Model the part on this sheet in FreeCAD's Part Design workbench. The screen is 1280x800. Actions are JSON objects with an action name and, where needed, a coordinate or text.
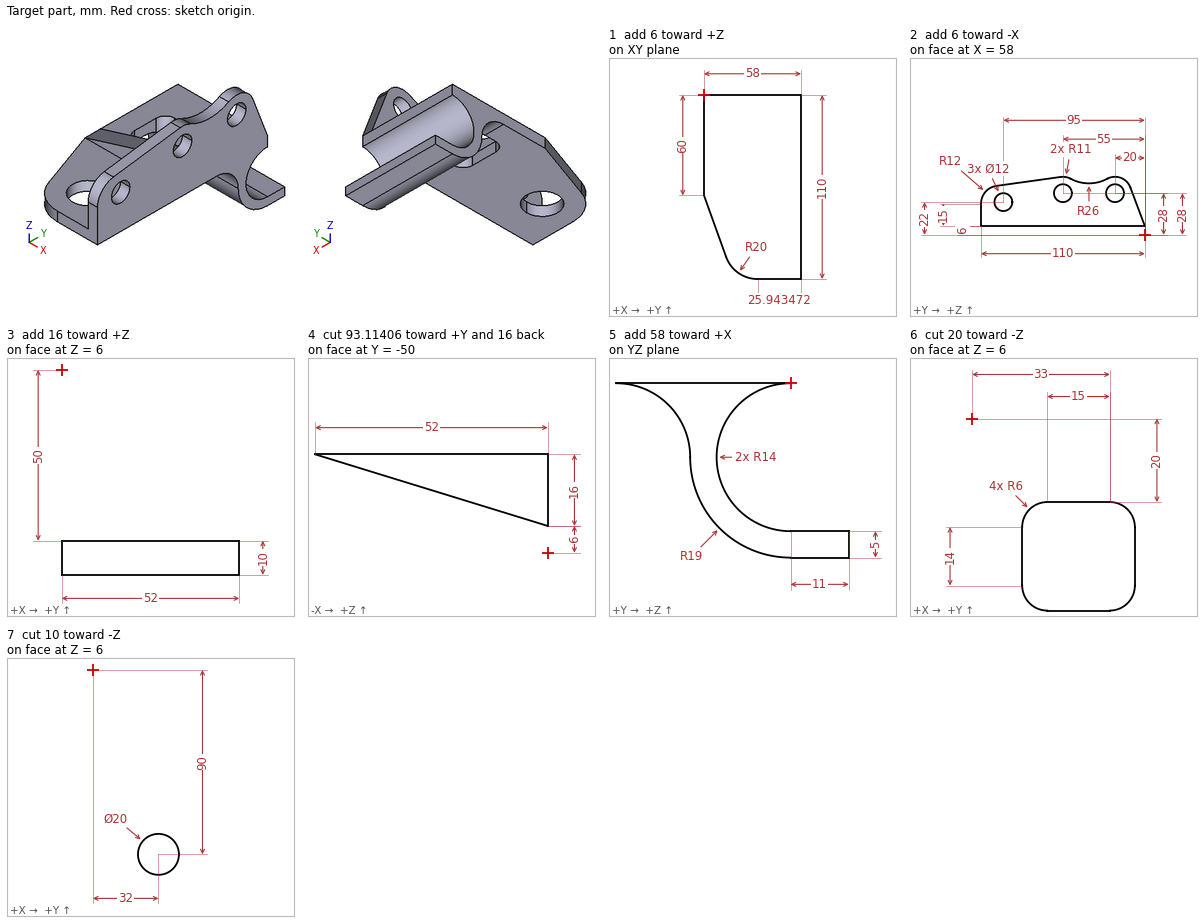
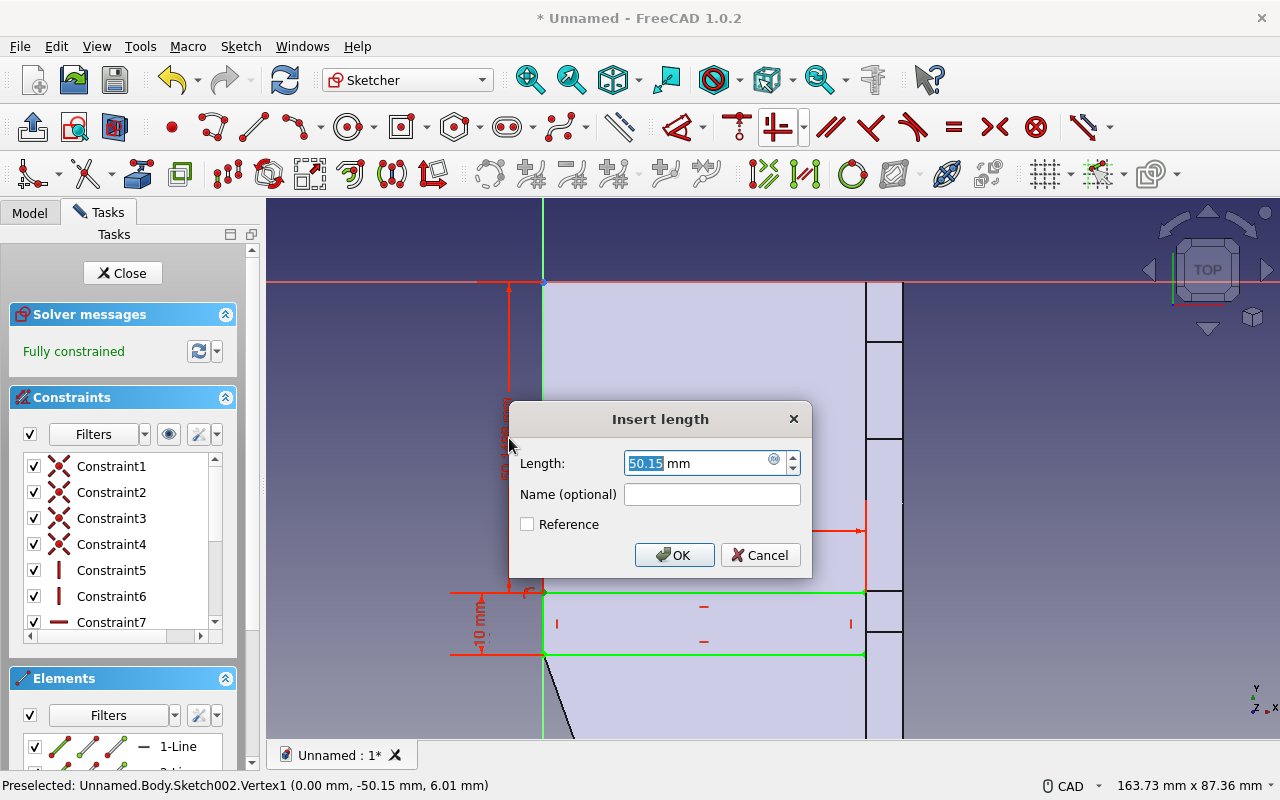
{"action": "type", "text": "50"}
{"action": "key", "text": "Return"}
{"action": "key", "text": "Escape"}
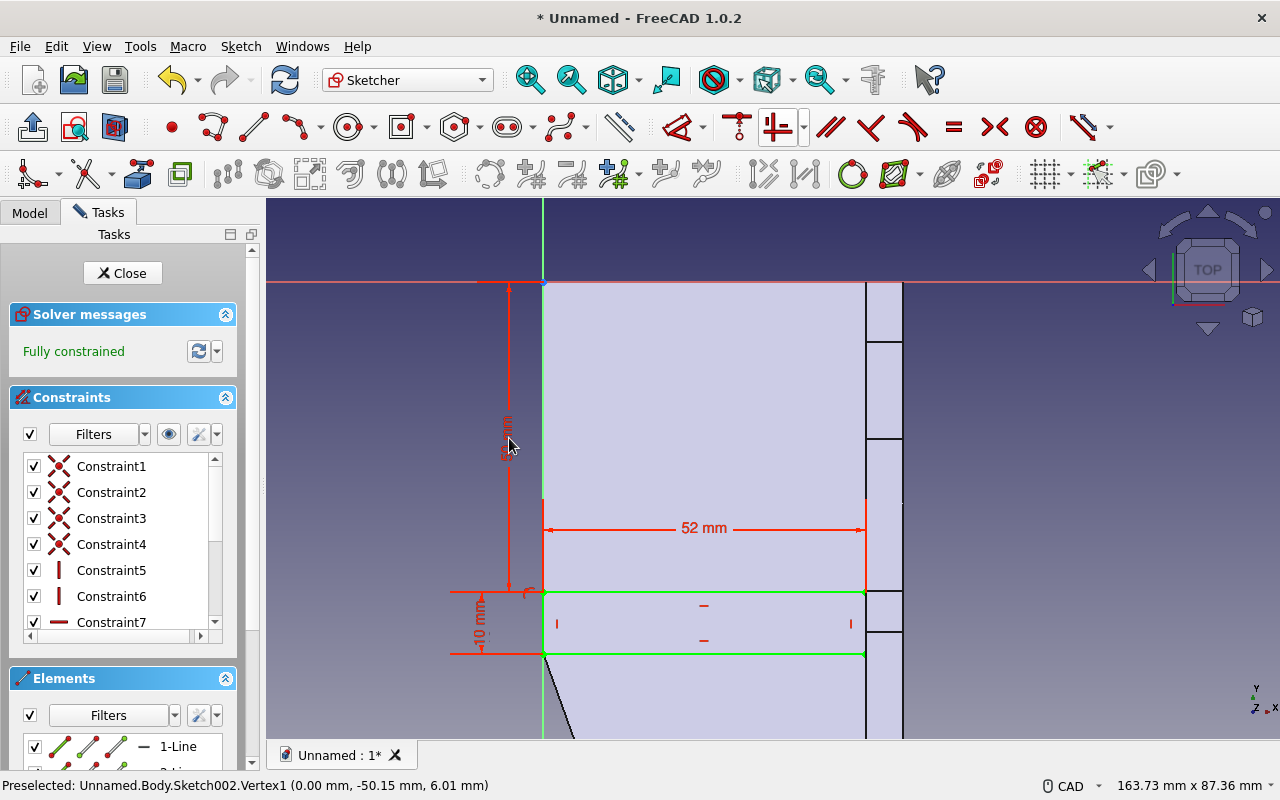
{"action": "left_click", "coordinate": [123, 273]}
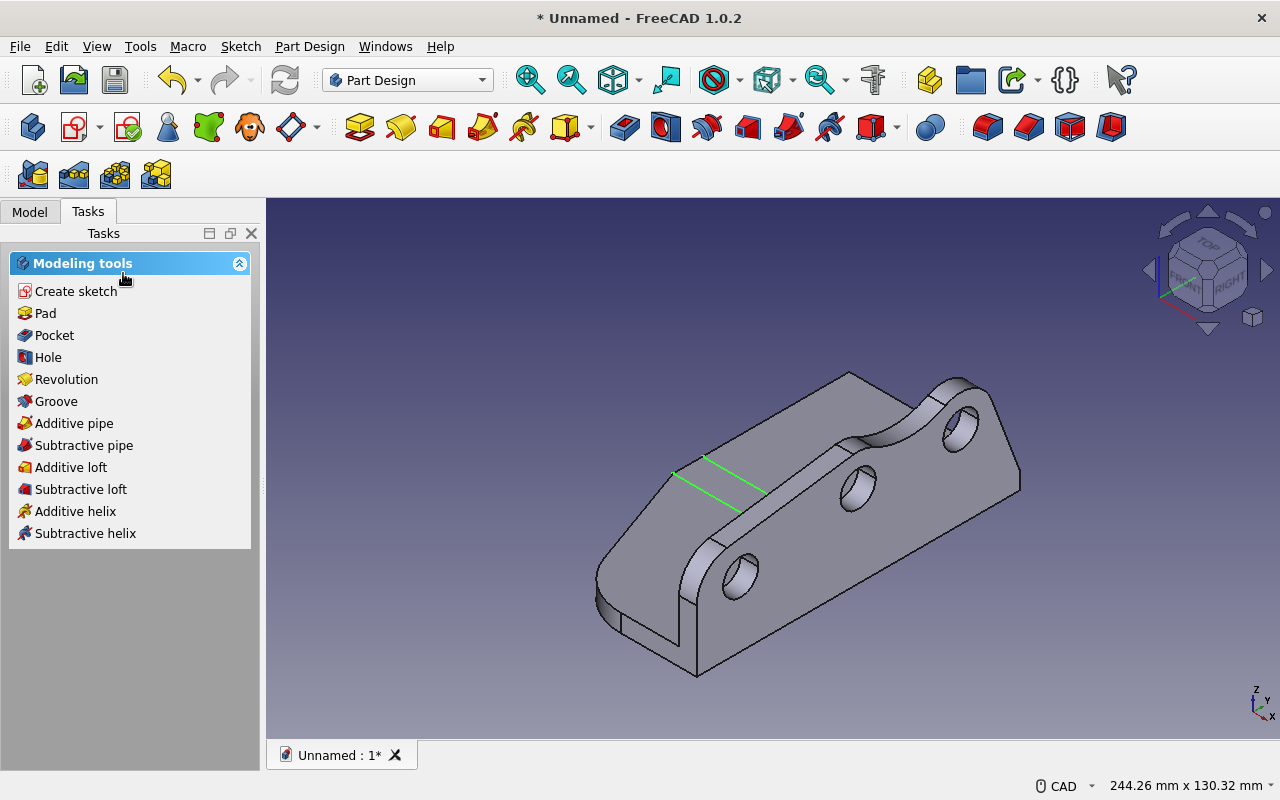
{"action": "left_click", "coordinate": [360, 128]}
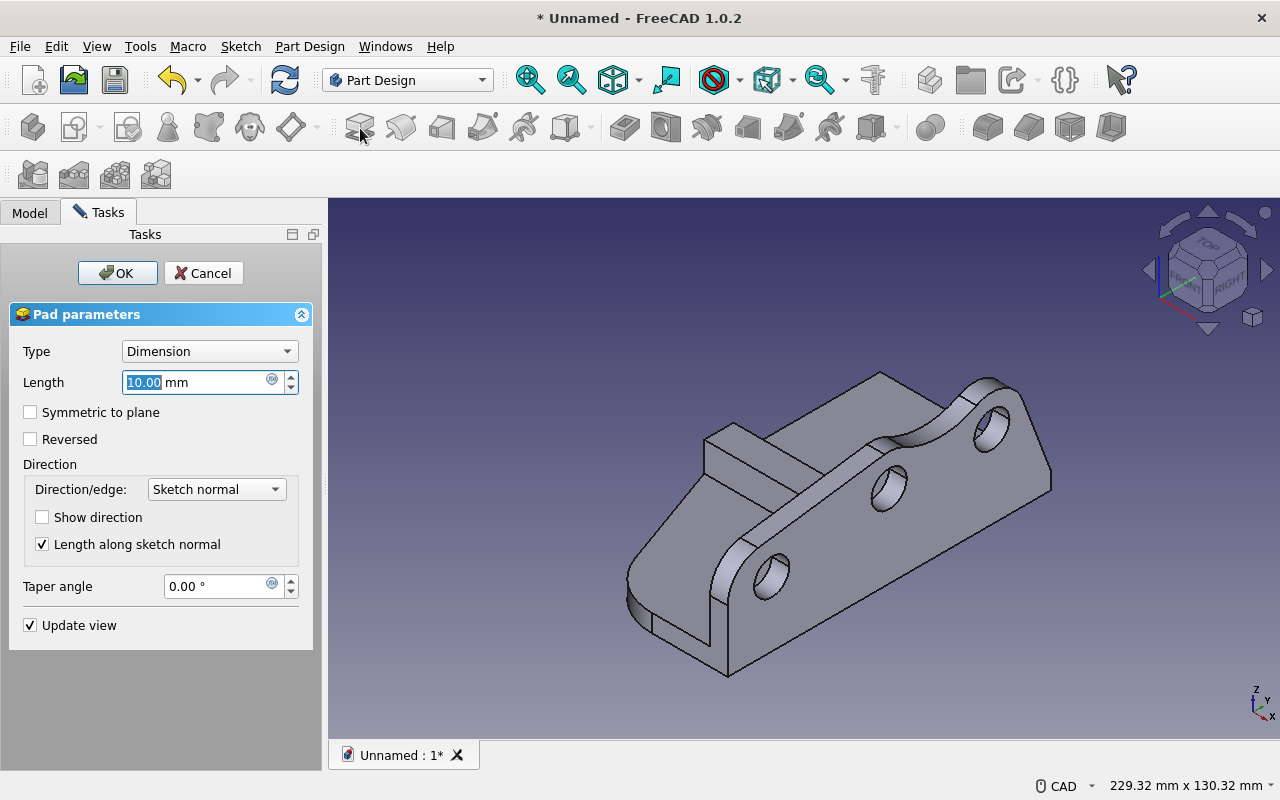
{"action": "type", "text": "16"}
{"action": "key", "text": "Tab"}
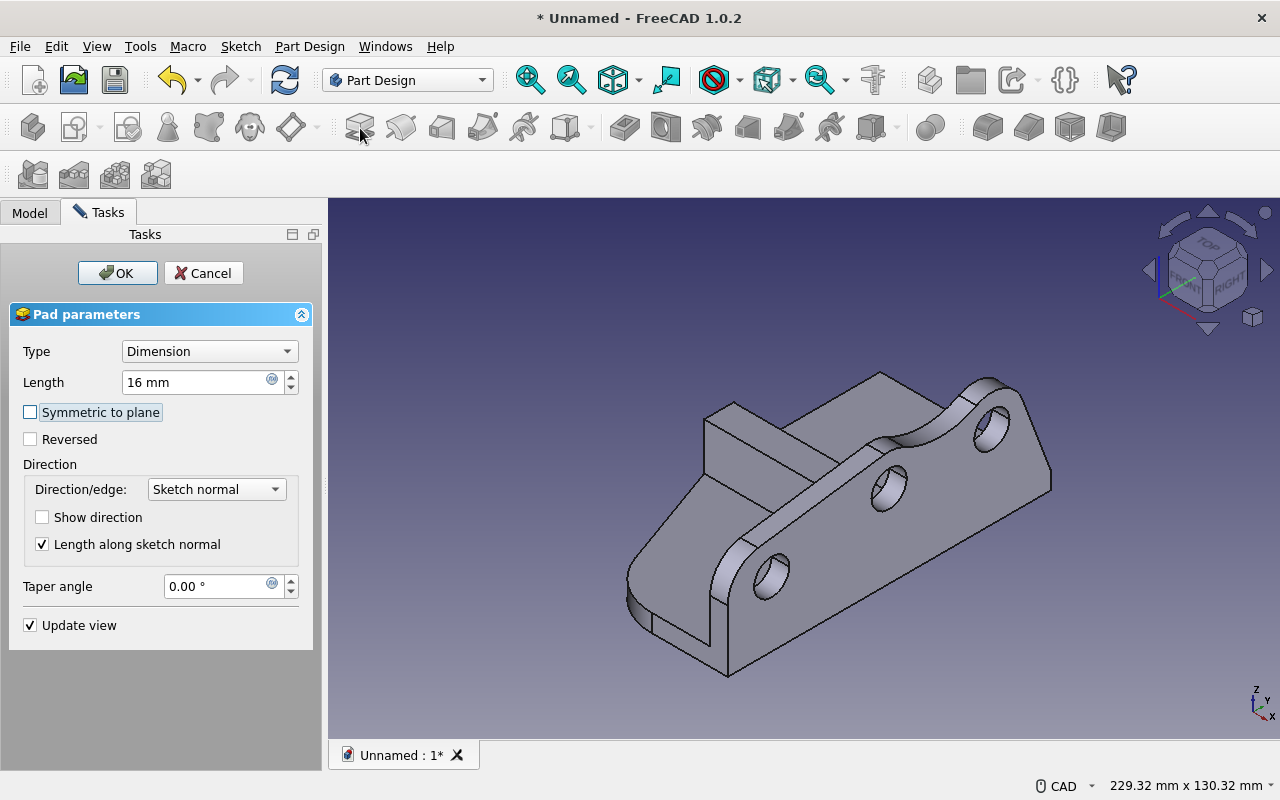
{"action": "left_click", "coordinate": [118, 273]}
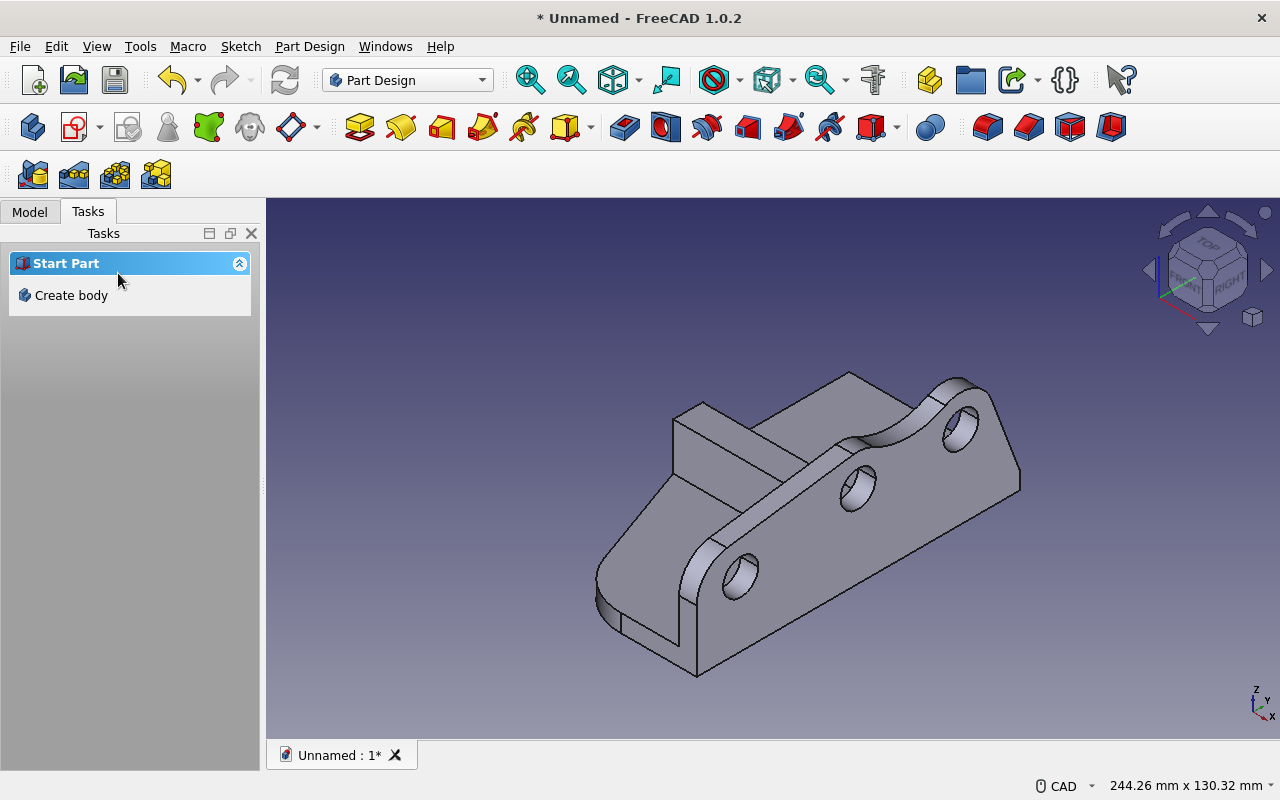
{"action": "key", "text": "4"}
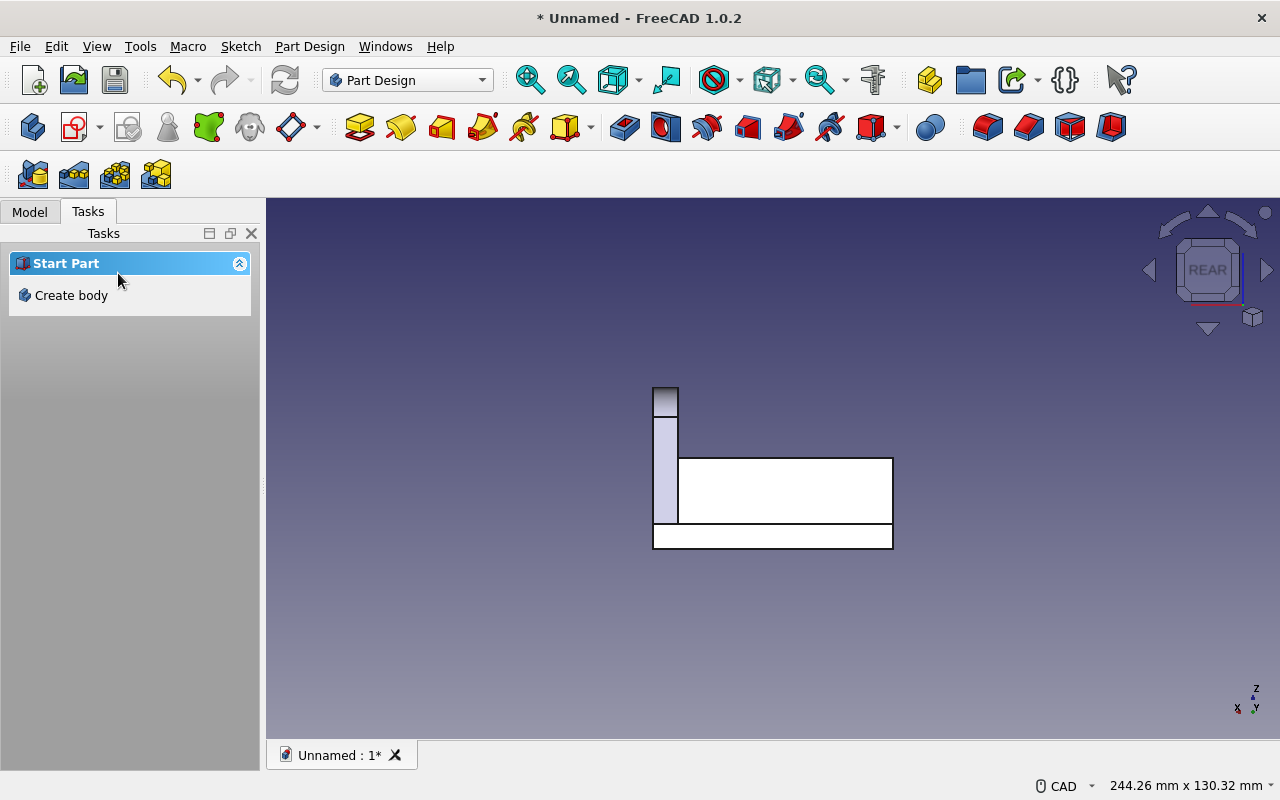
{"action": "left_click", "coordinate": [531, 80]}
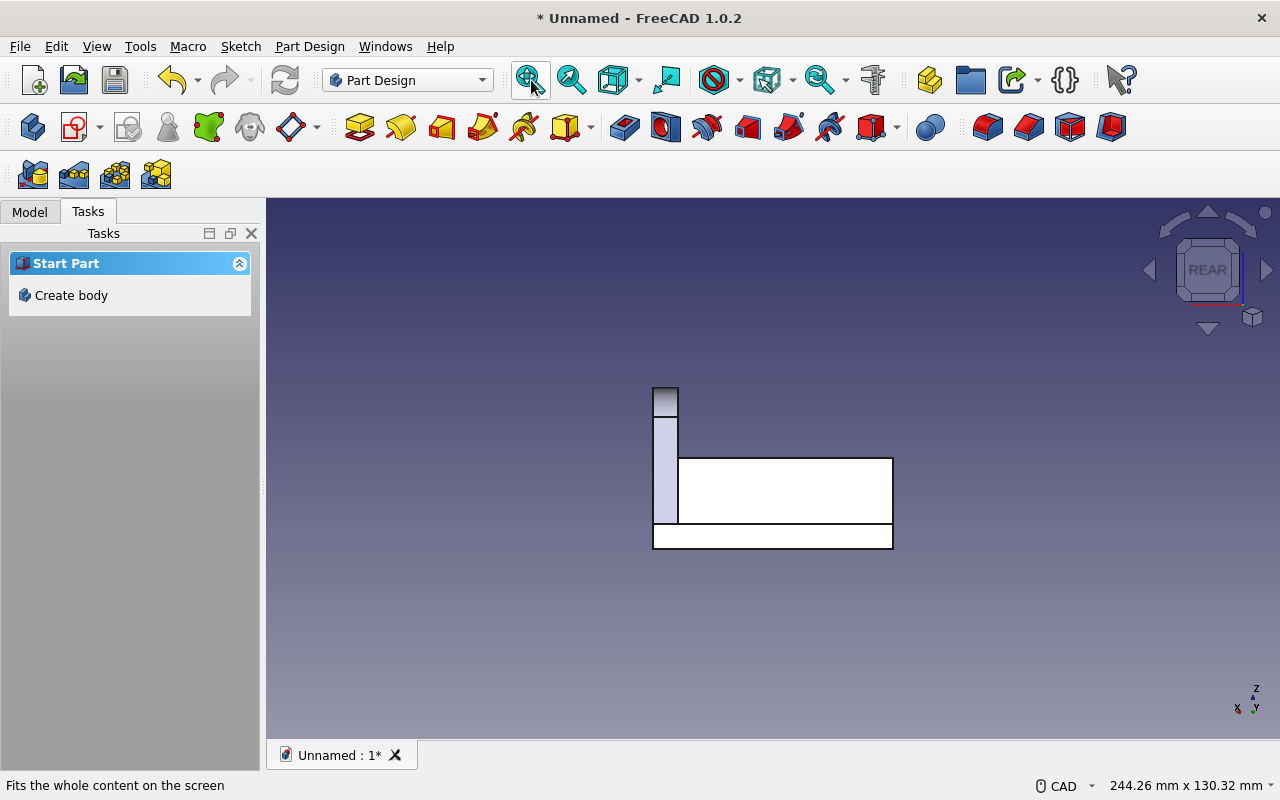
{"action": "left_click", "coordinate": [724, 490]}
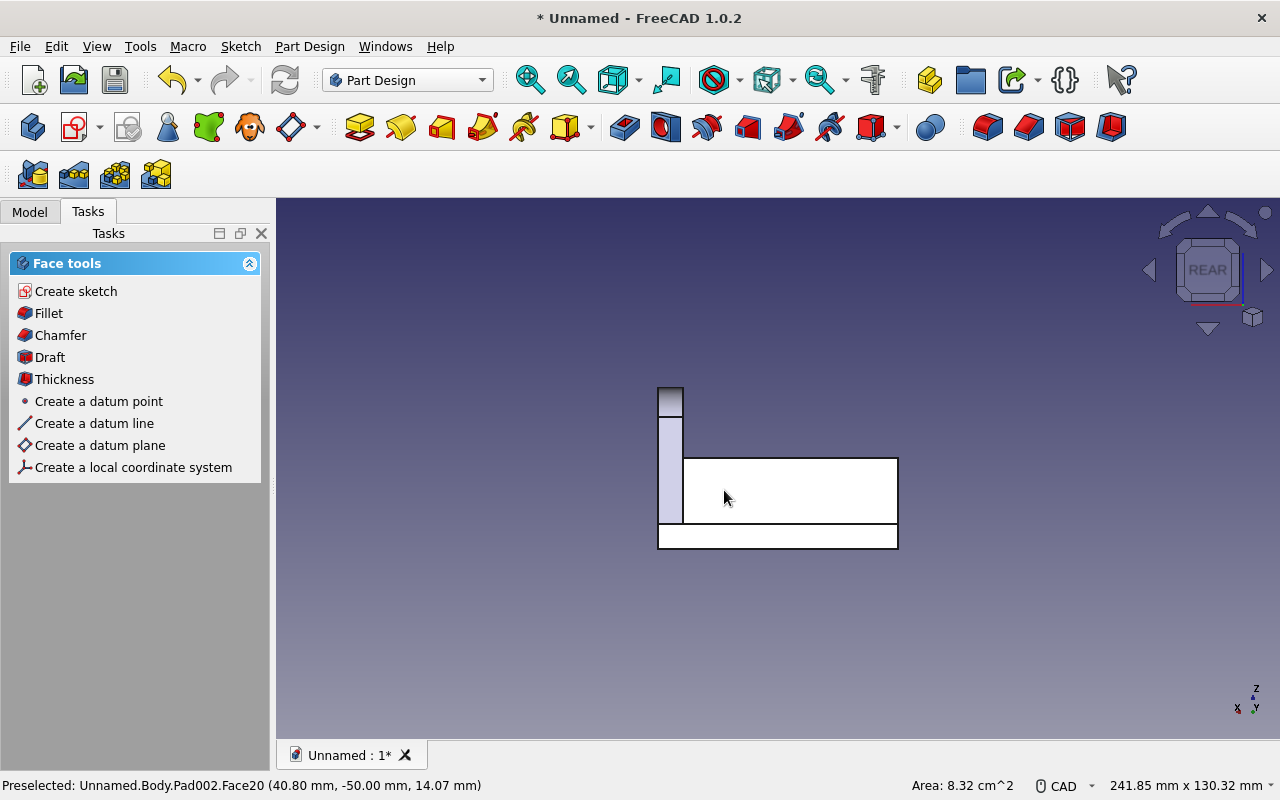
{"action": "left_click", "coordinate": [74, 128]}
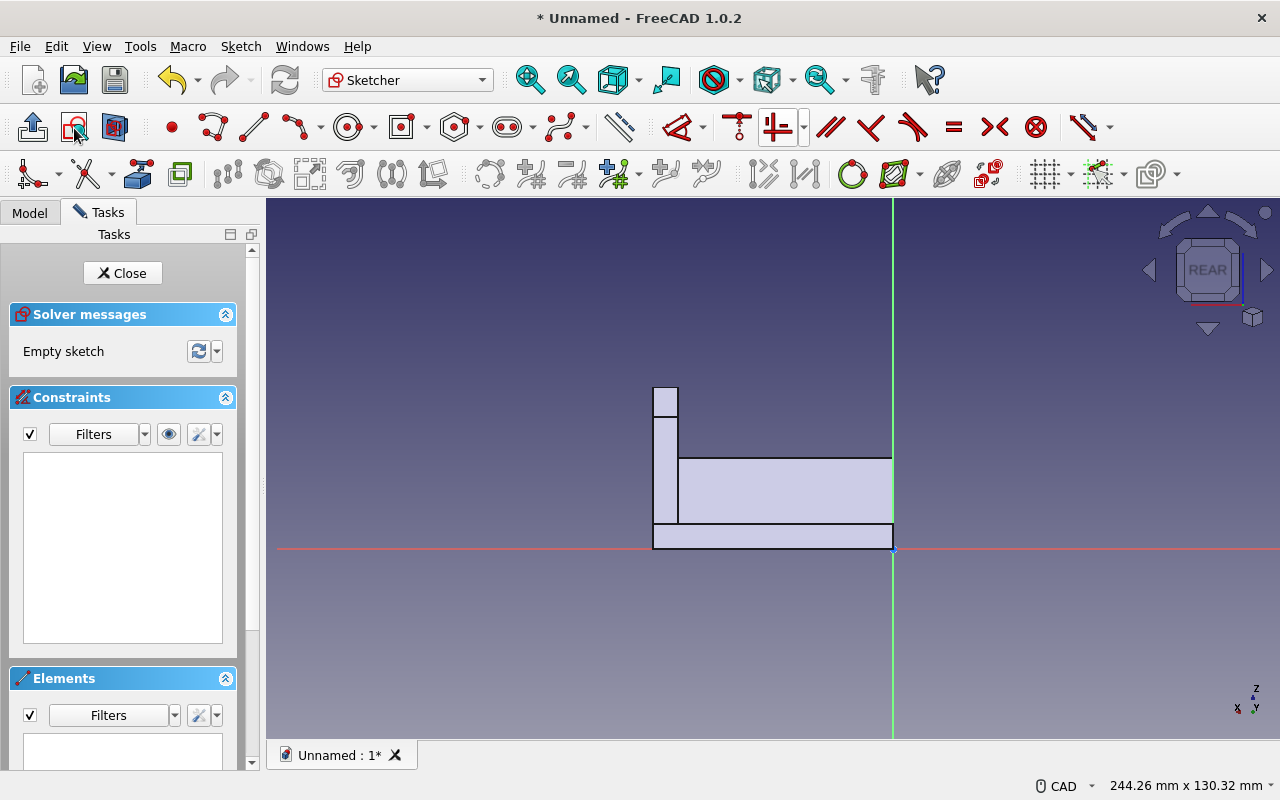
{"action": "key", "text": "q s"}